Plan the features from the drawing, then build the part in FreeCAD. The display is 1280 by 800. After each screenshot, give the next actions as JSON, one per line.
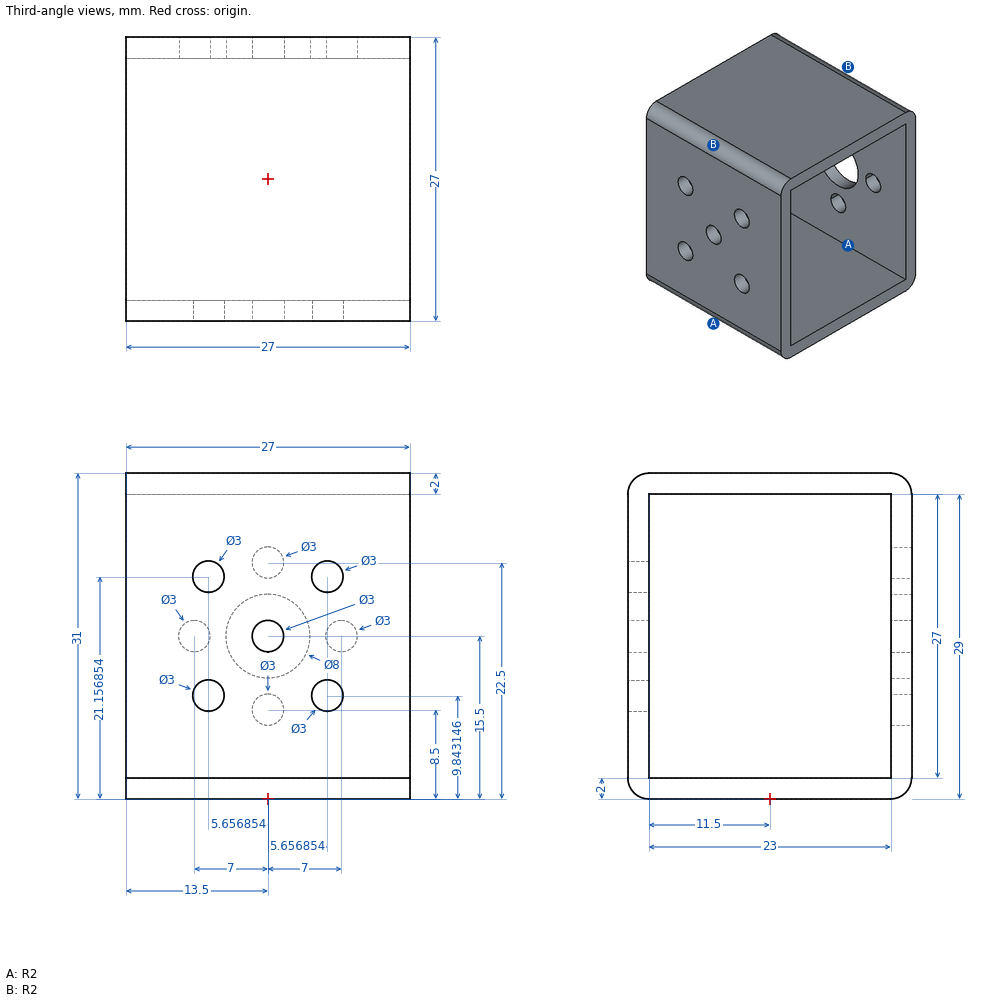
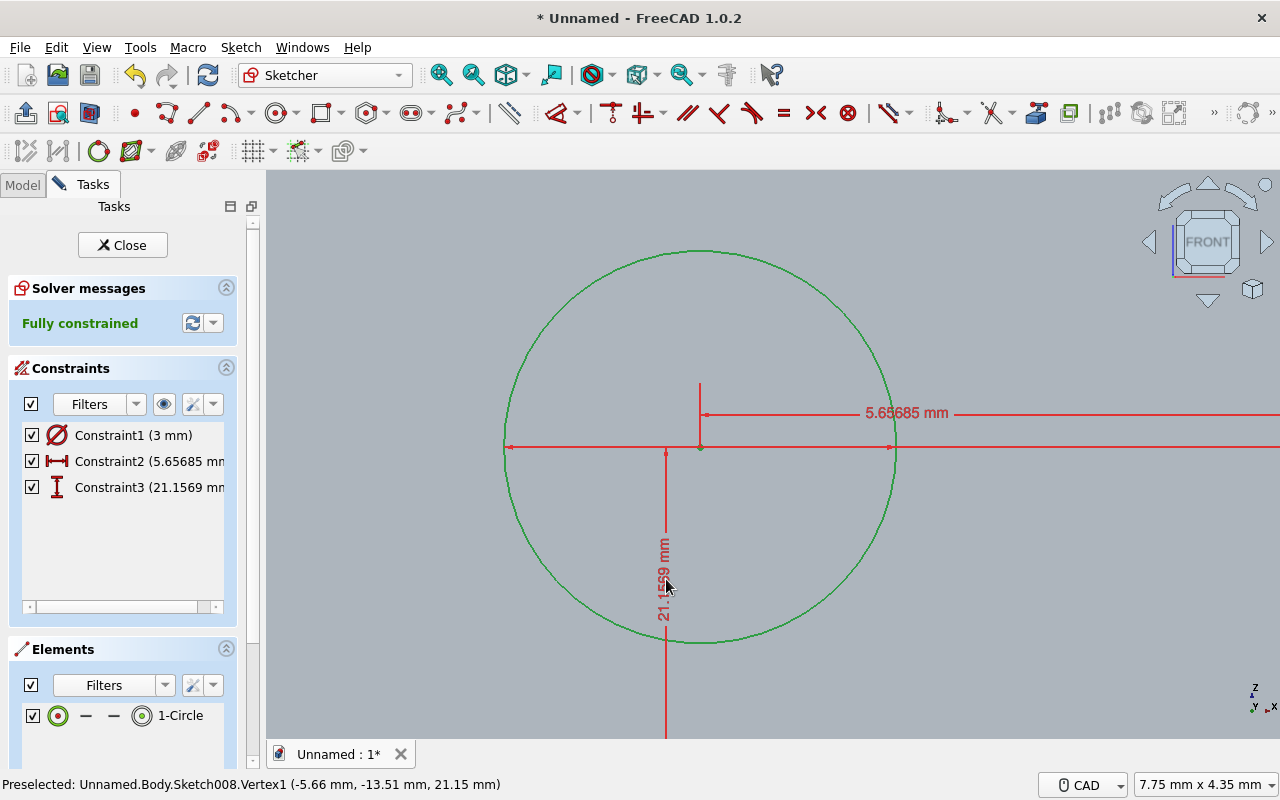
{"action": "left_click", "coordinate": [123, 245]}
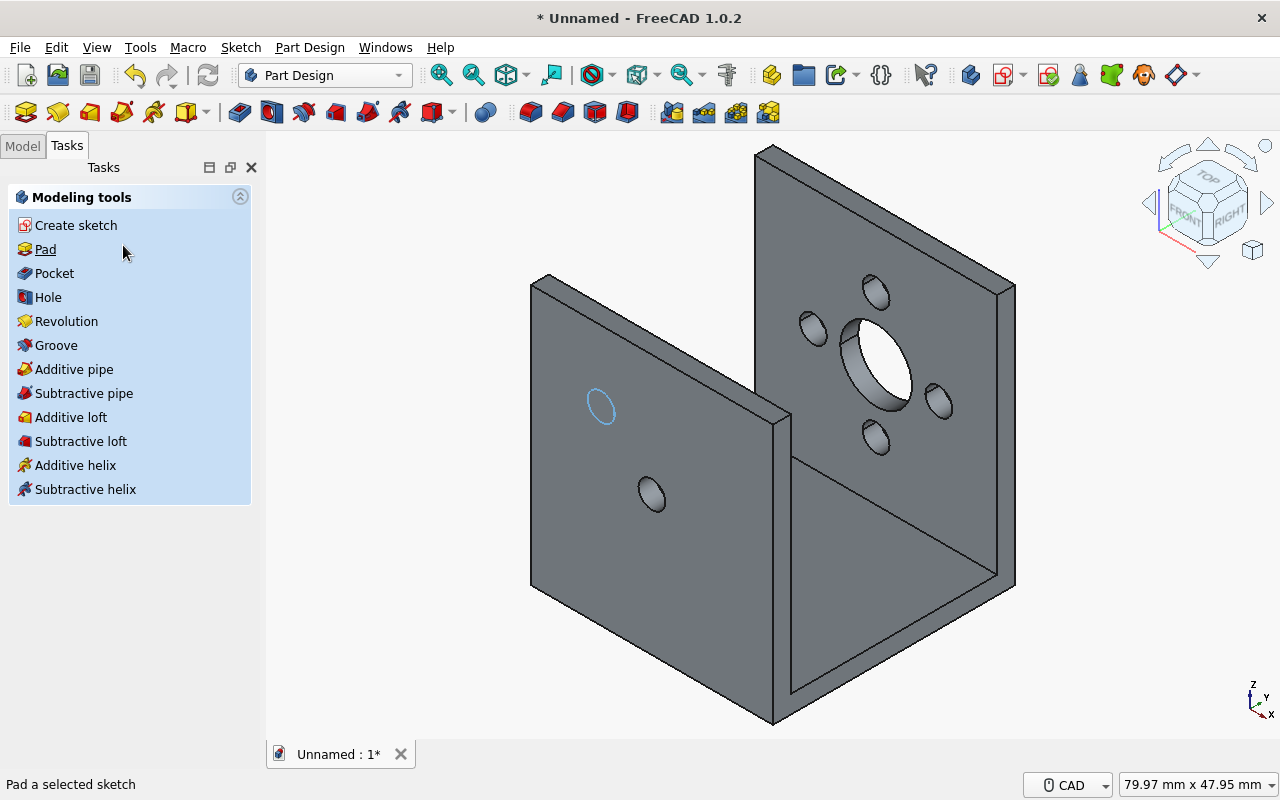
{"action": "left_click", "coordinate": [240, 112]}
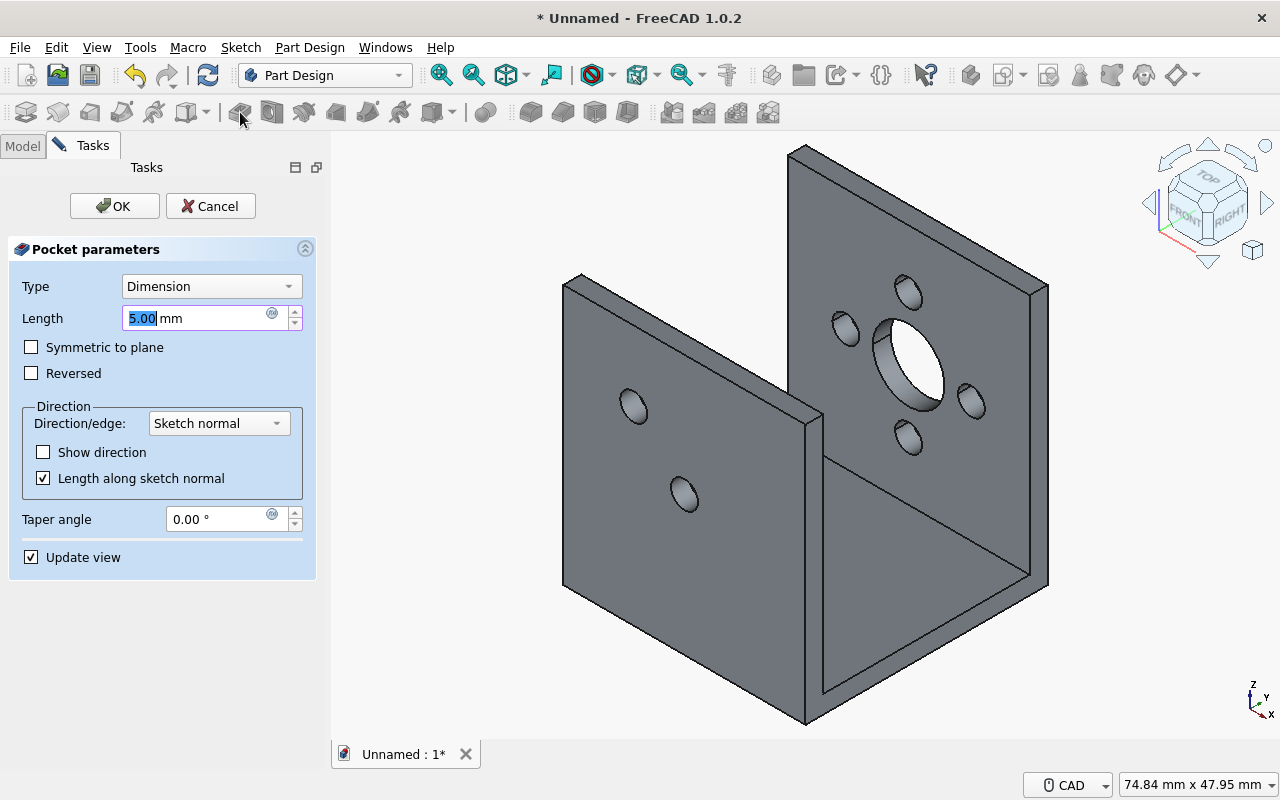
{"action": "left_click", "coordinate": [212, 286]}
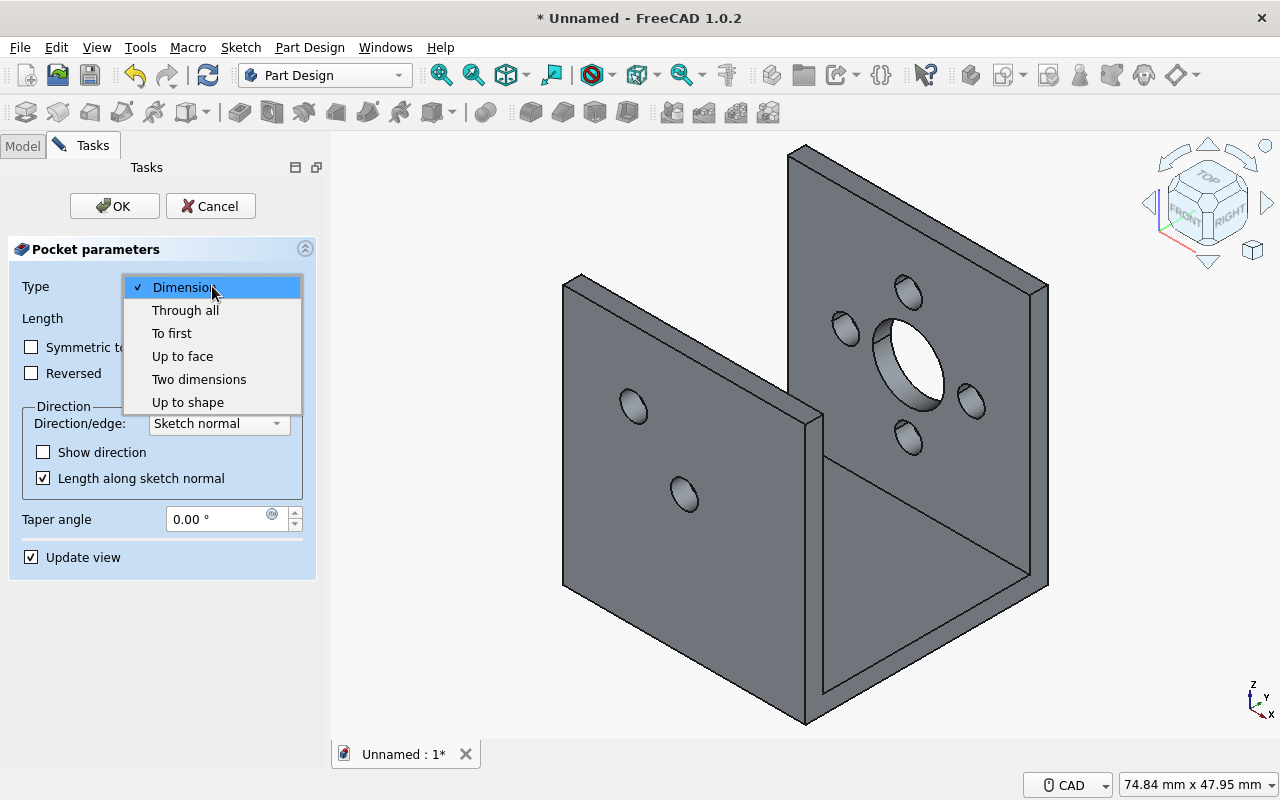
{"action": "left_click", "coordinate": [212, 334]}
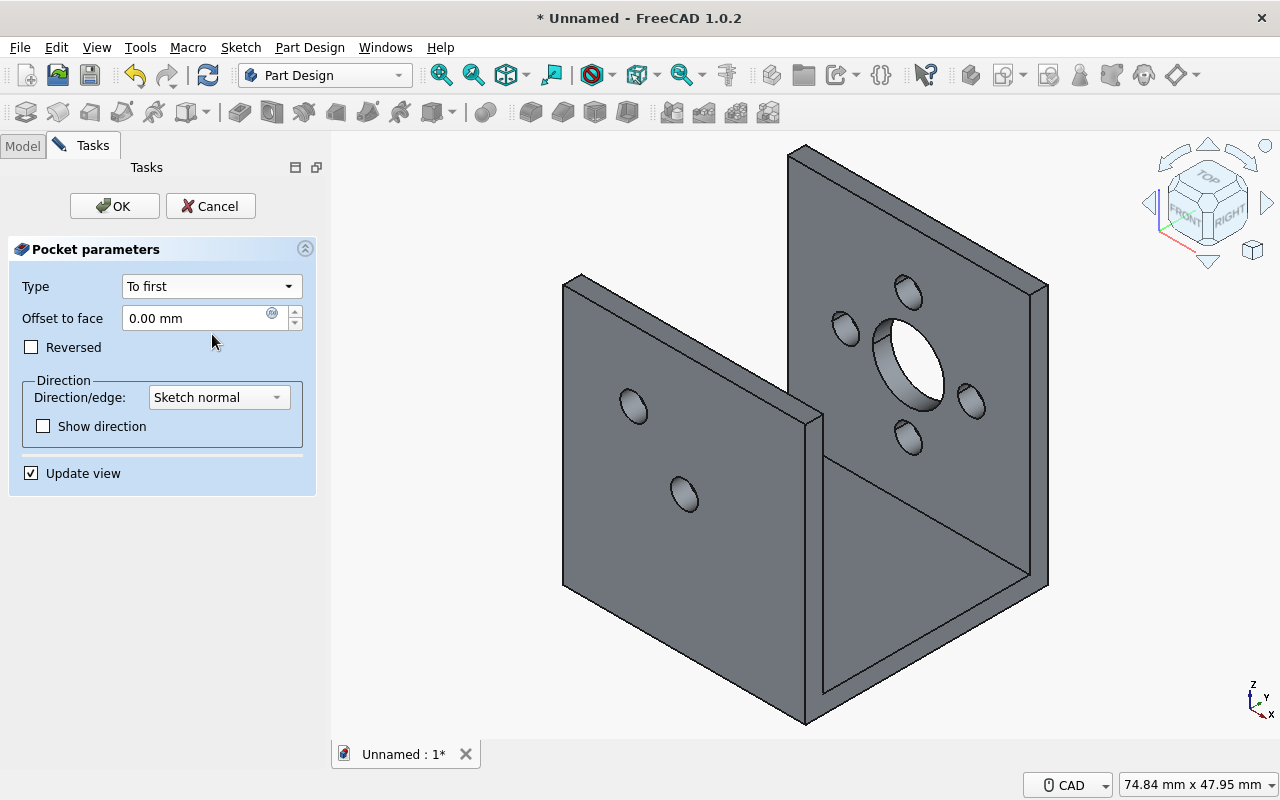
{"action": "left_click", "coordinate": [115, 206]}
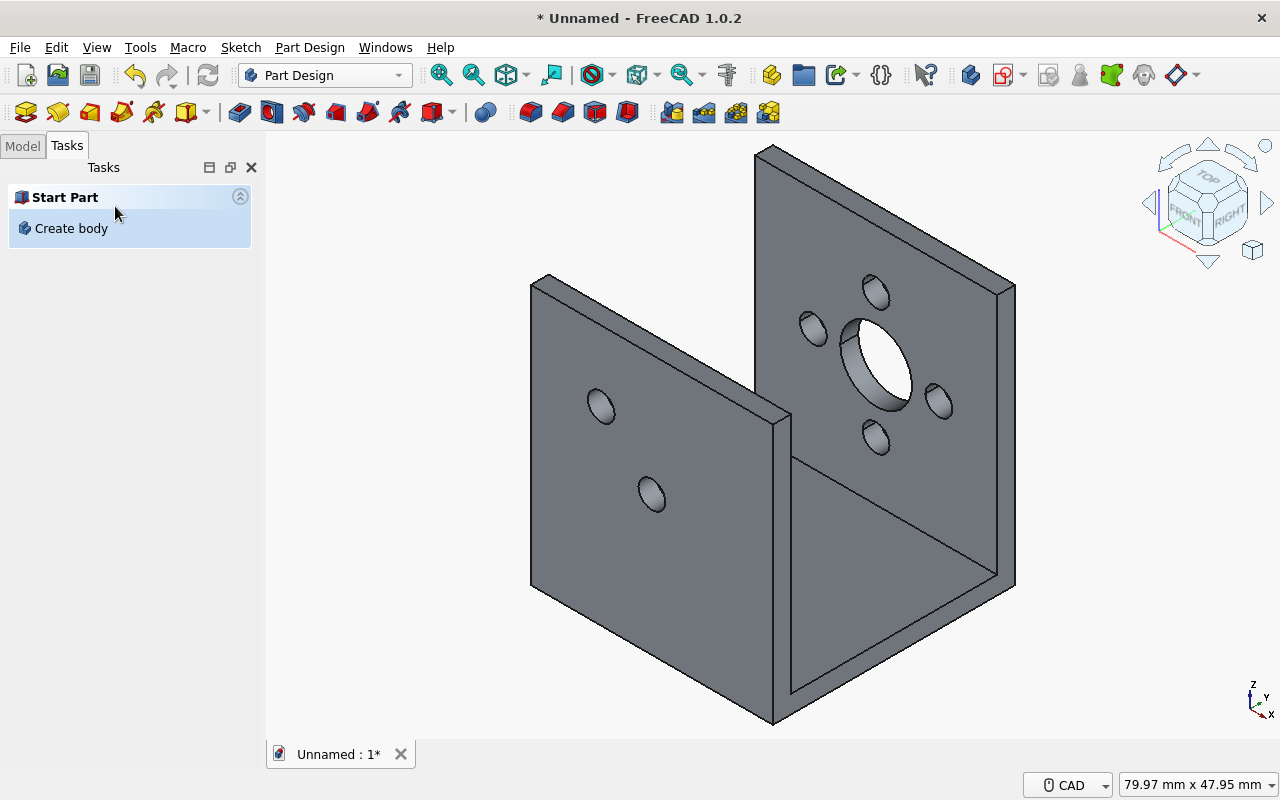
{"action": "left_click", "coordinate": [687, 438]}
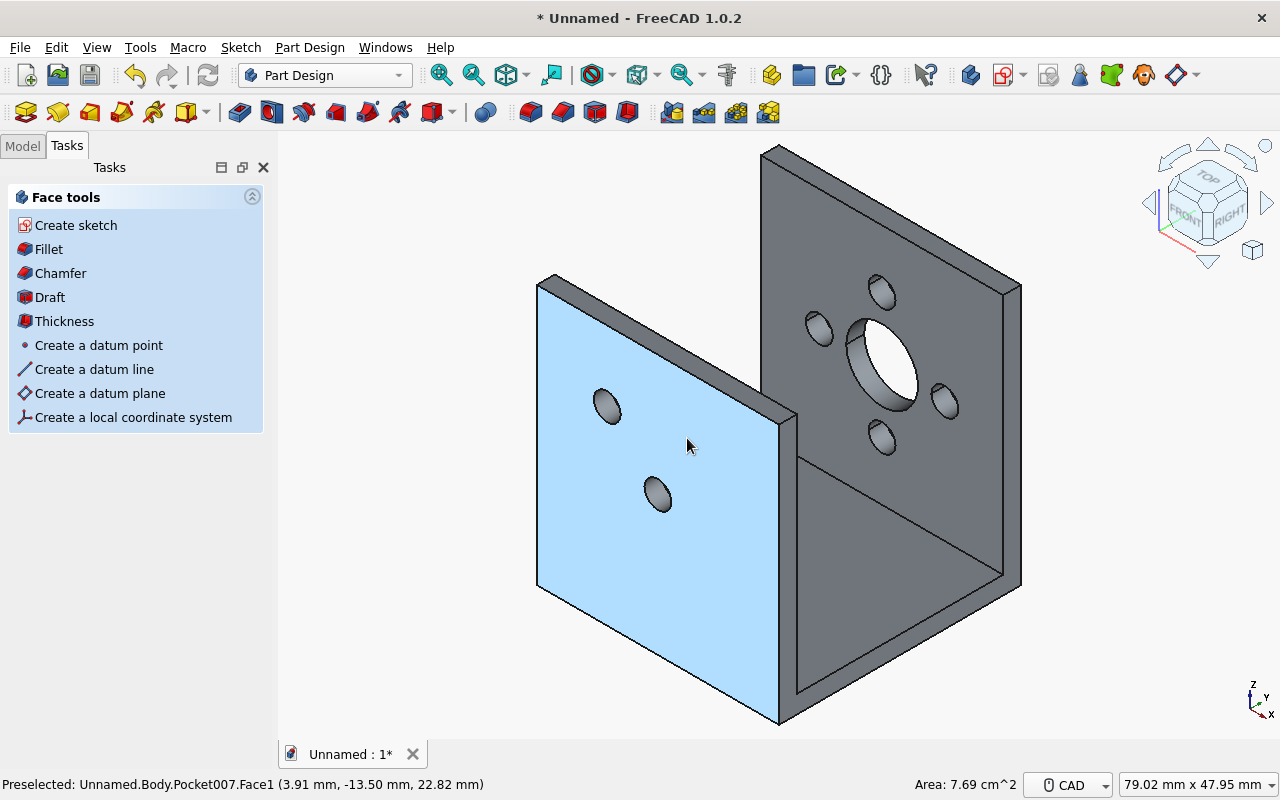
{"action": "left_click", "coordinate": [1004, 76]}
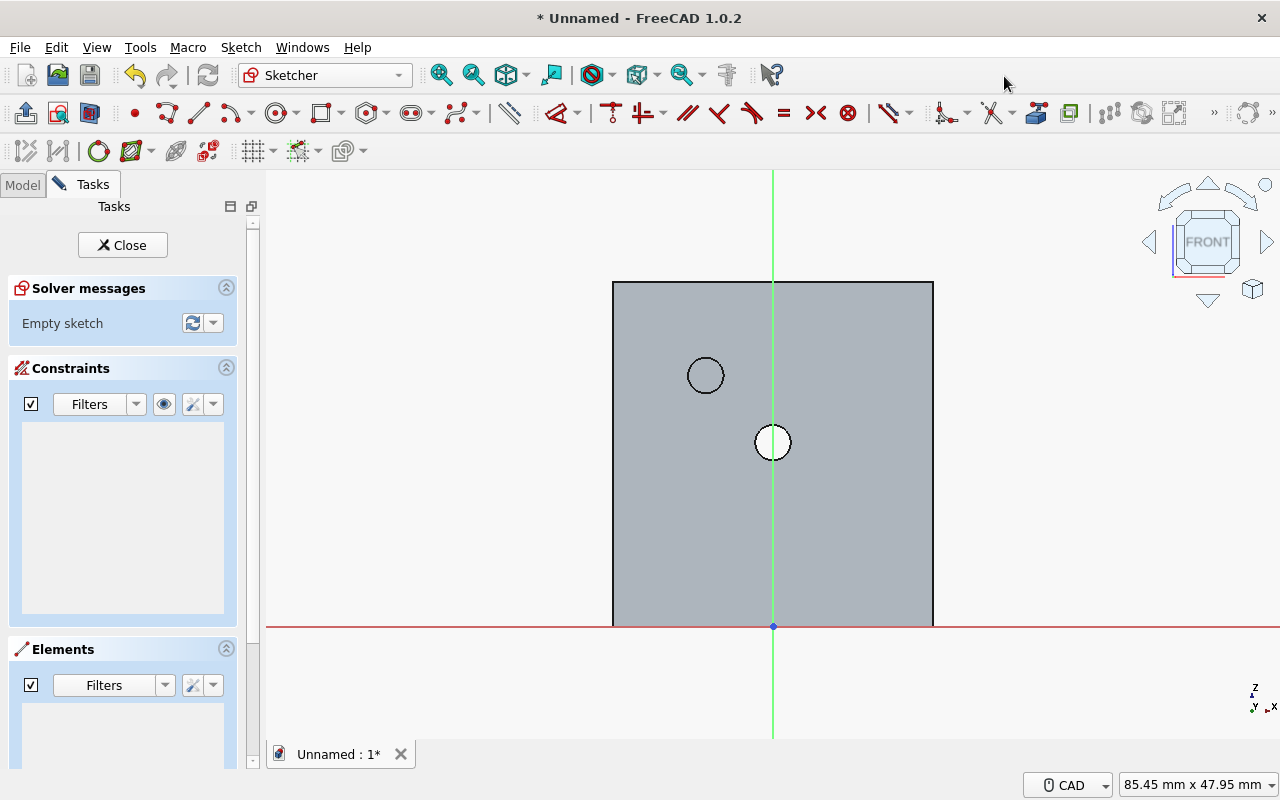
{"action": "scroll", "coordinate": [854, 368], "scroll_direction": "up", "scroll_amount": 12}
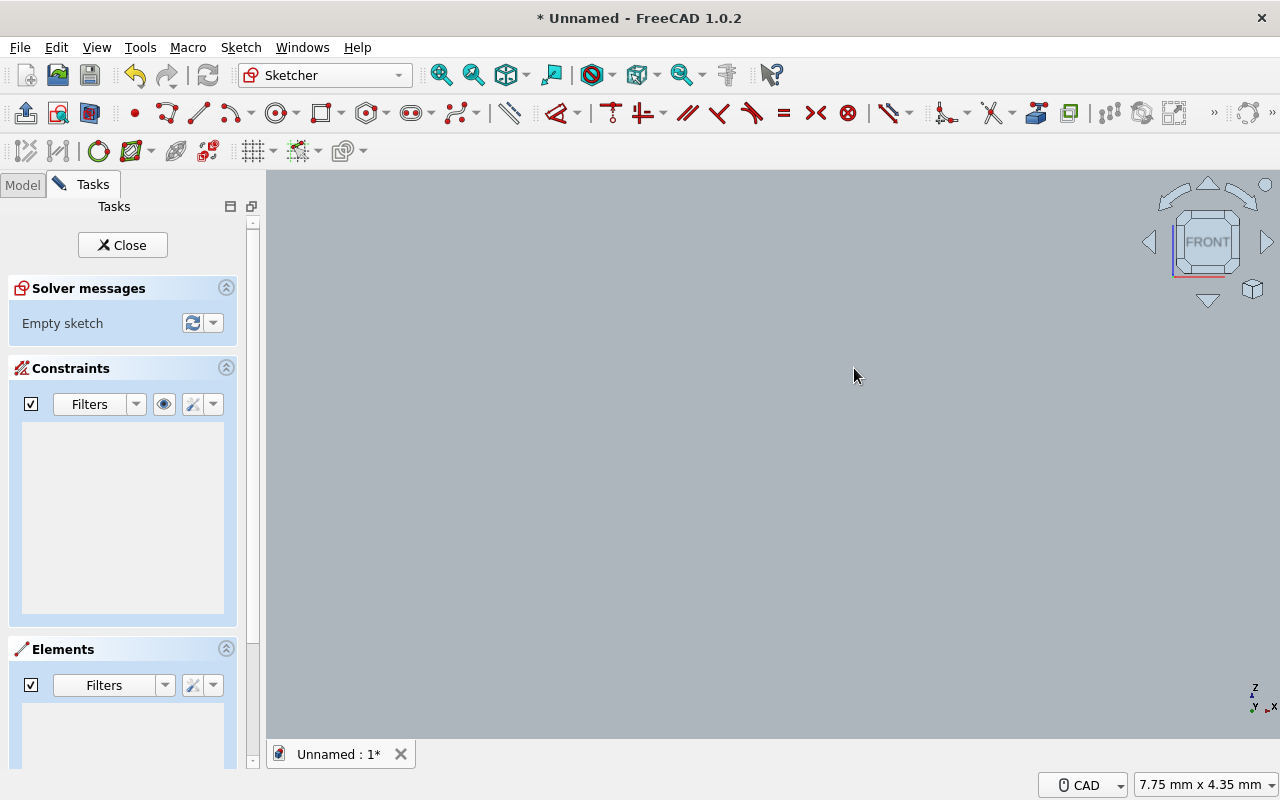
{"action": "left_click", "coordinate": [276, 114]}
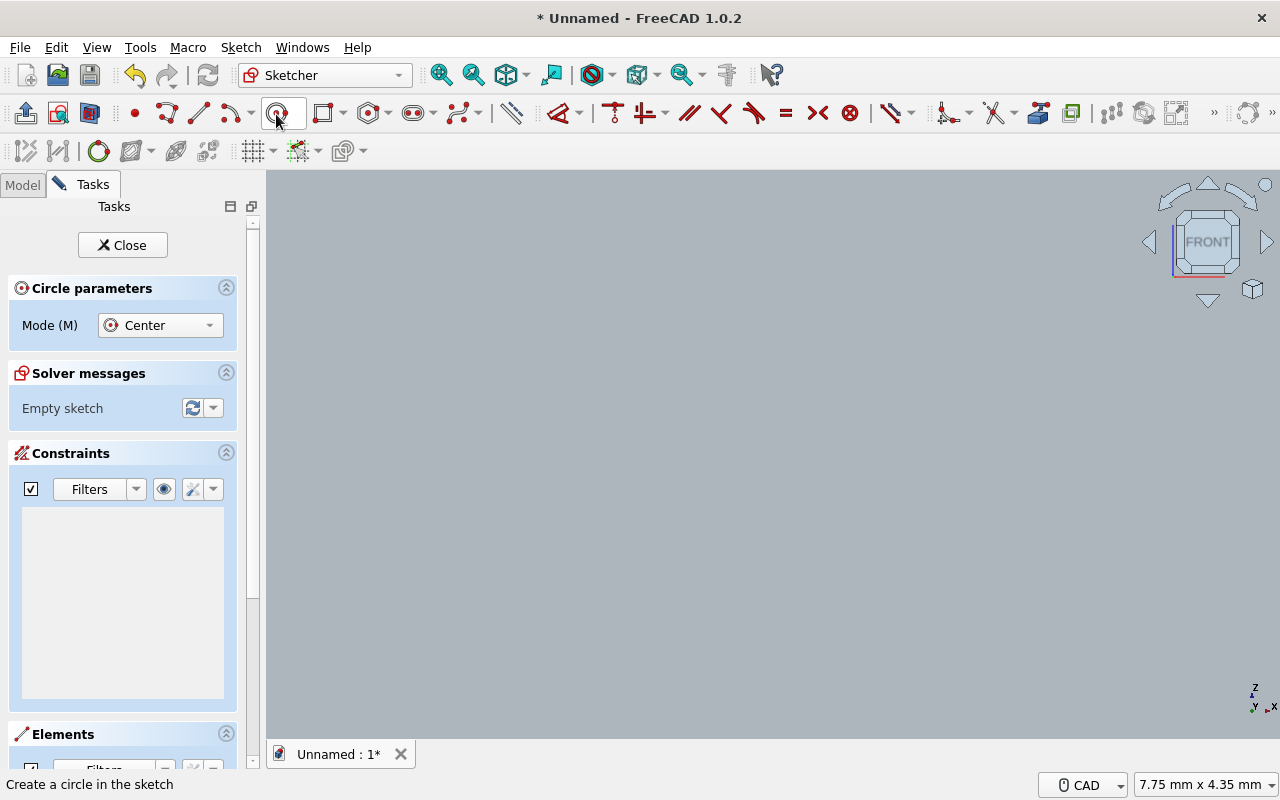
{"action": "left_click", "coordinate": [695, 447]}
{"action": "mouse_move", "coordinate": [834, 308]}